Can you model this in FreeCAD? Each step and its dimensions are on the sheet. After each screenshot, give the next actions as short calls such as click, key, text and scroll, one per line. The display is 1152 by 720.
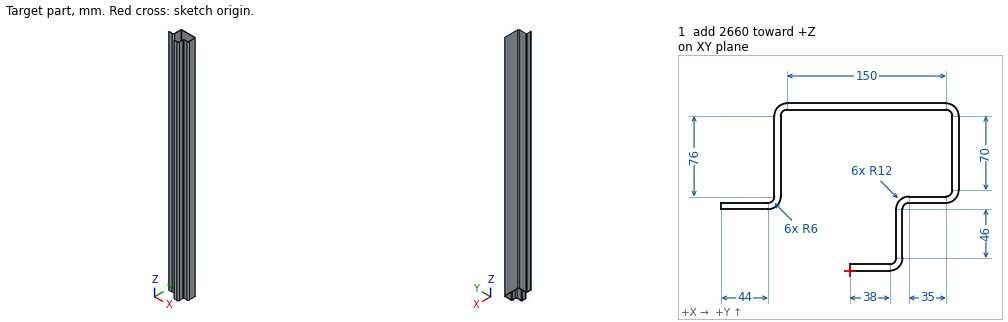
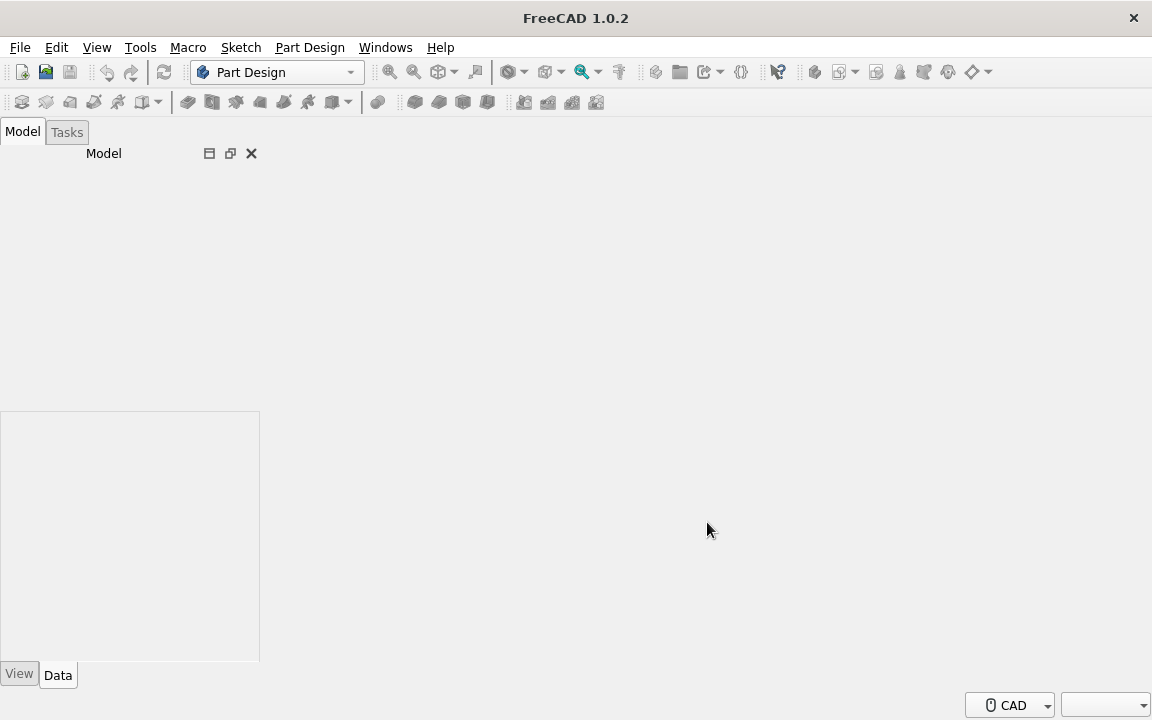
key(ctrl+n)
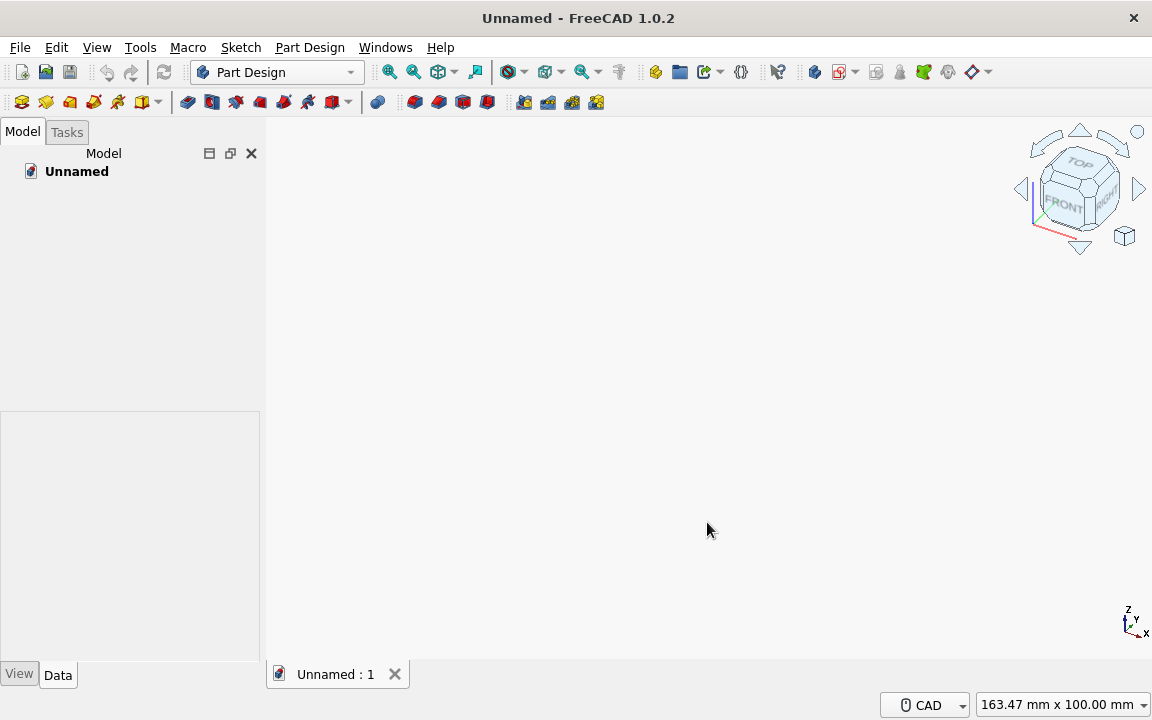
click(840, 72)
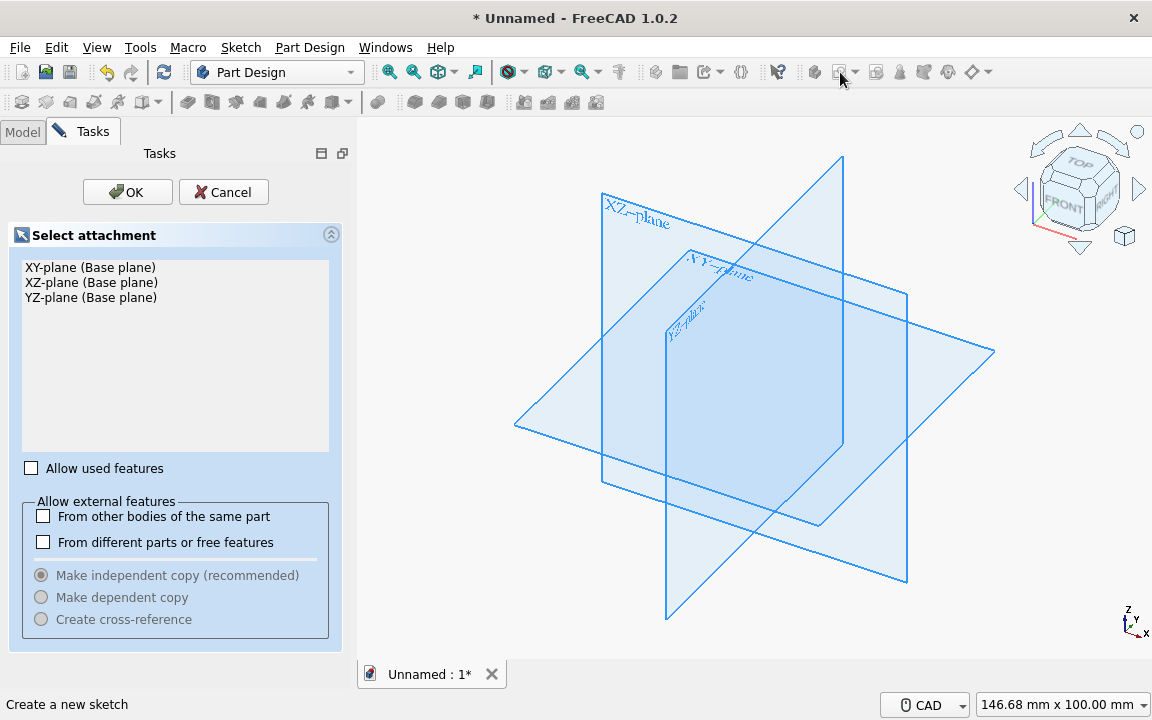
click(82, 268)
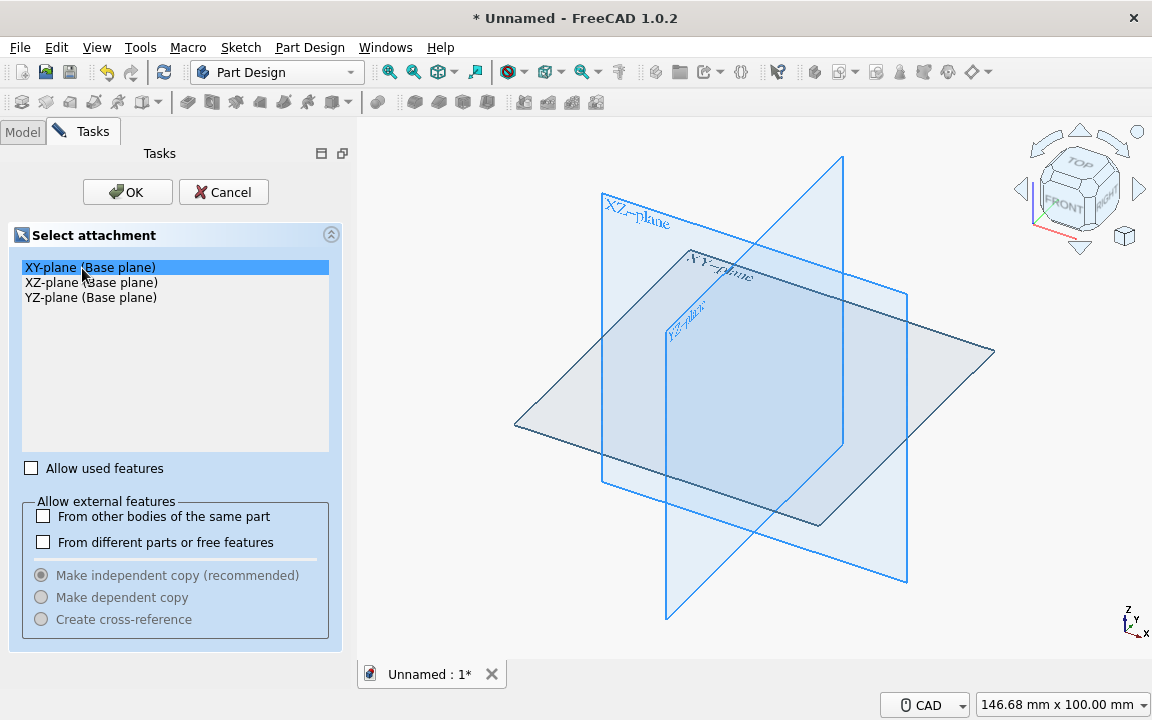
click(128, 192)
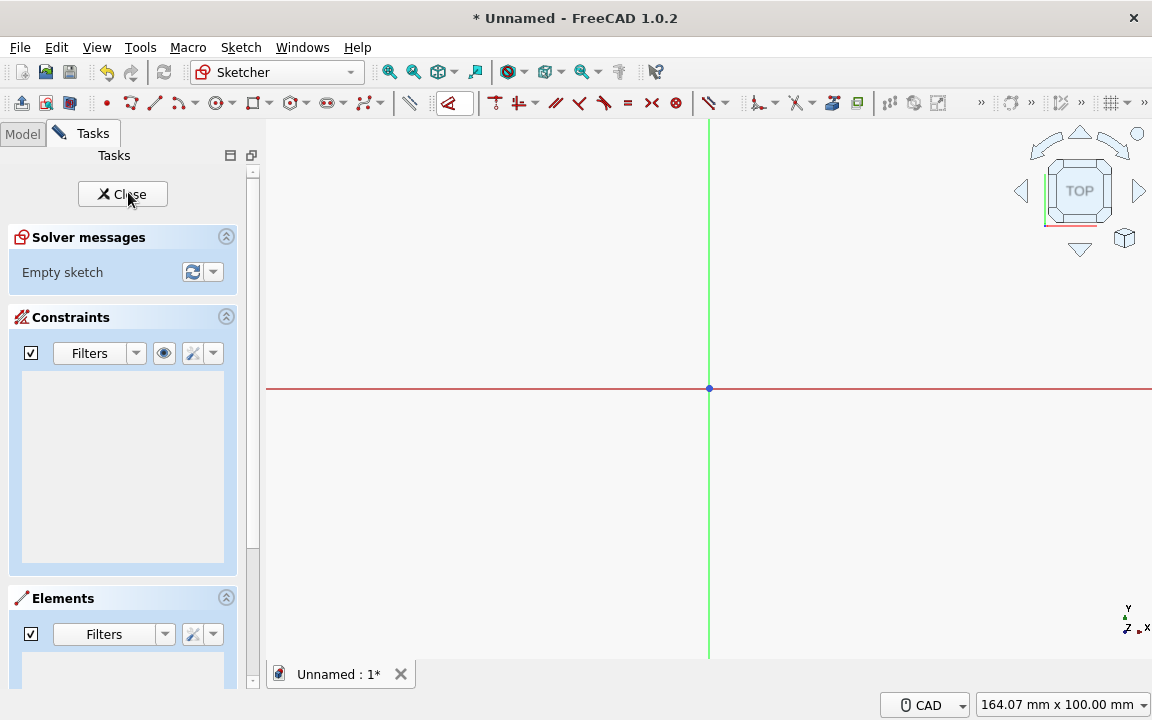
scroll(629, 631, down, 5)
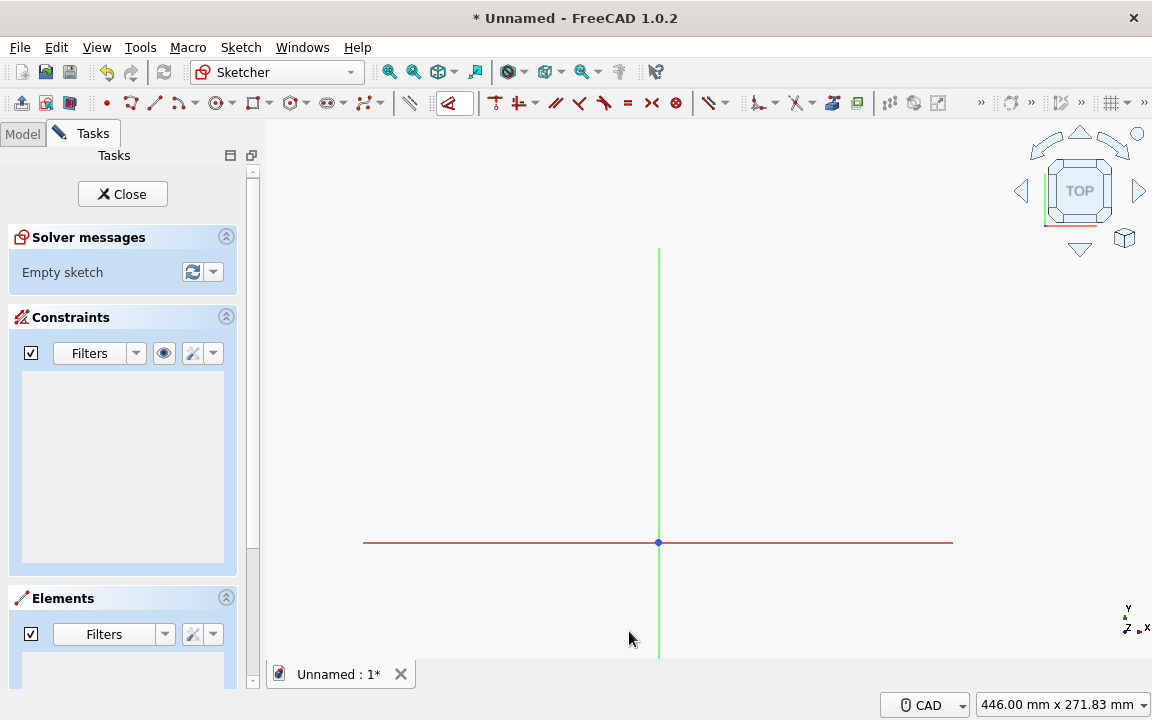
key(g)
key(l)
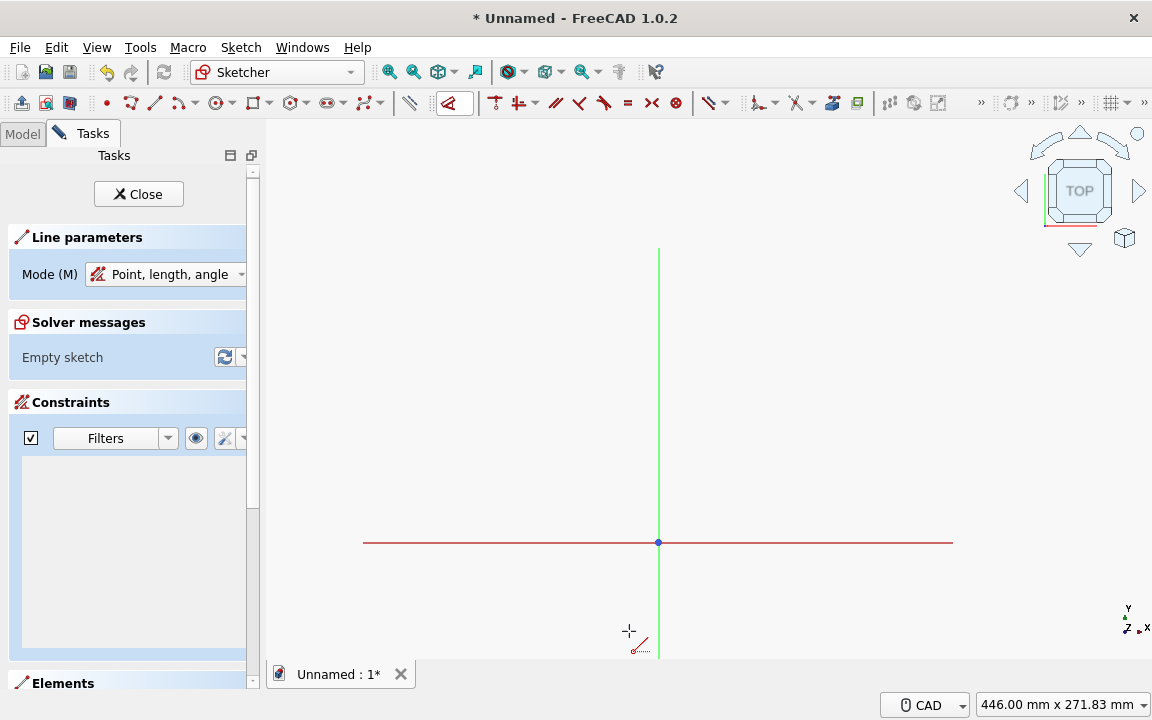
click(518, 253)
click(518, 404)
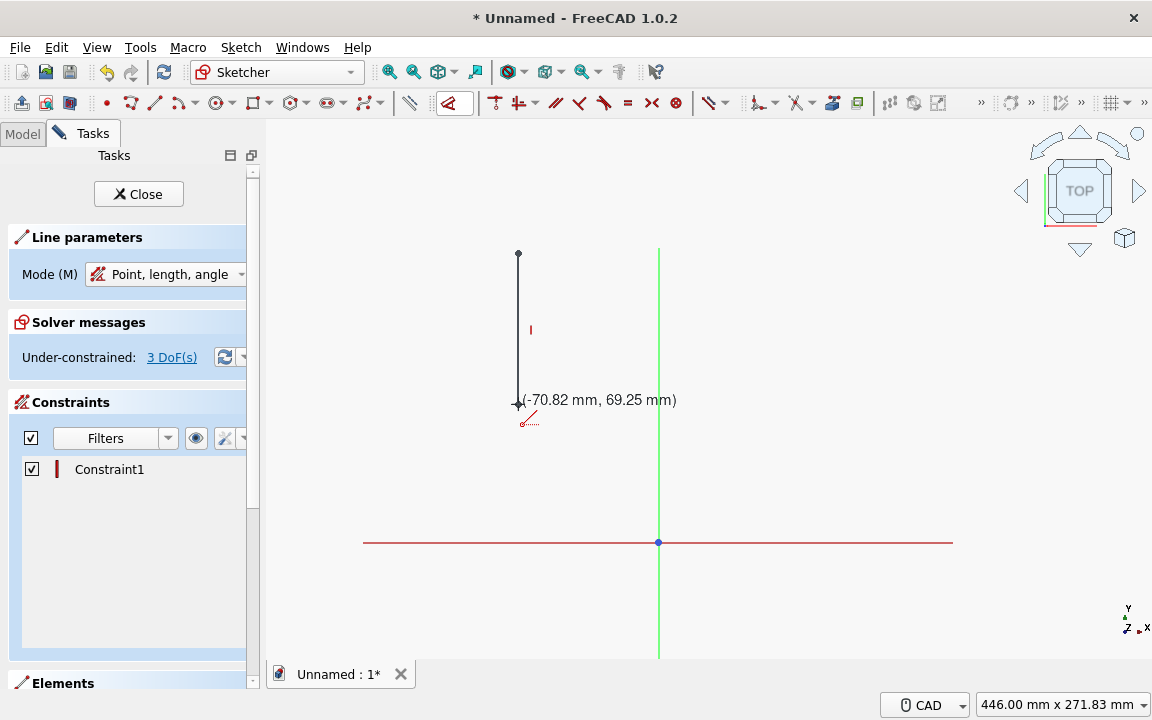
click(132, 104)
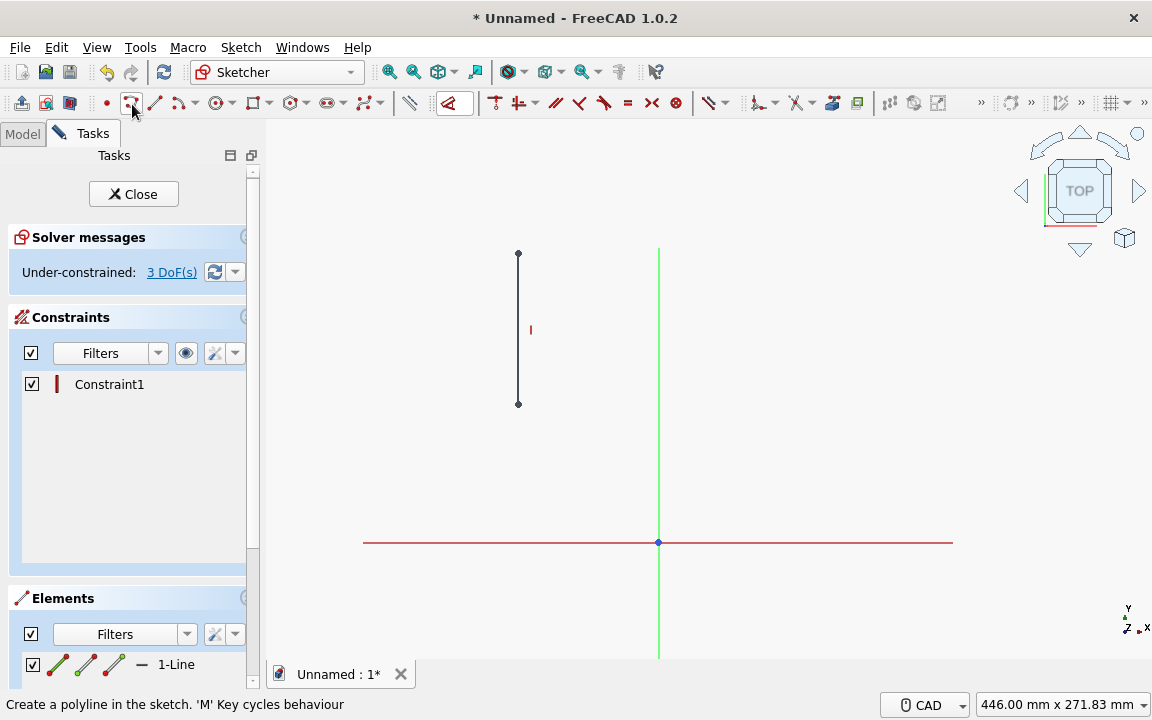
click(506, 415)
click(418, 415)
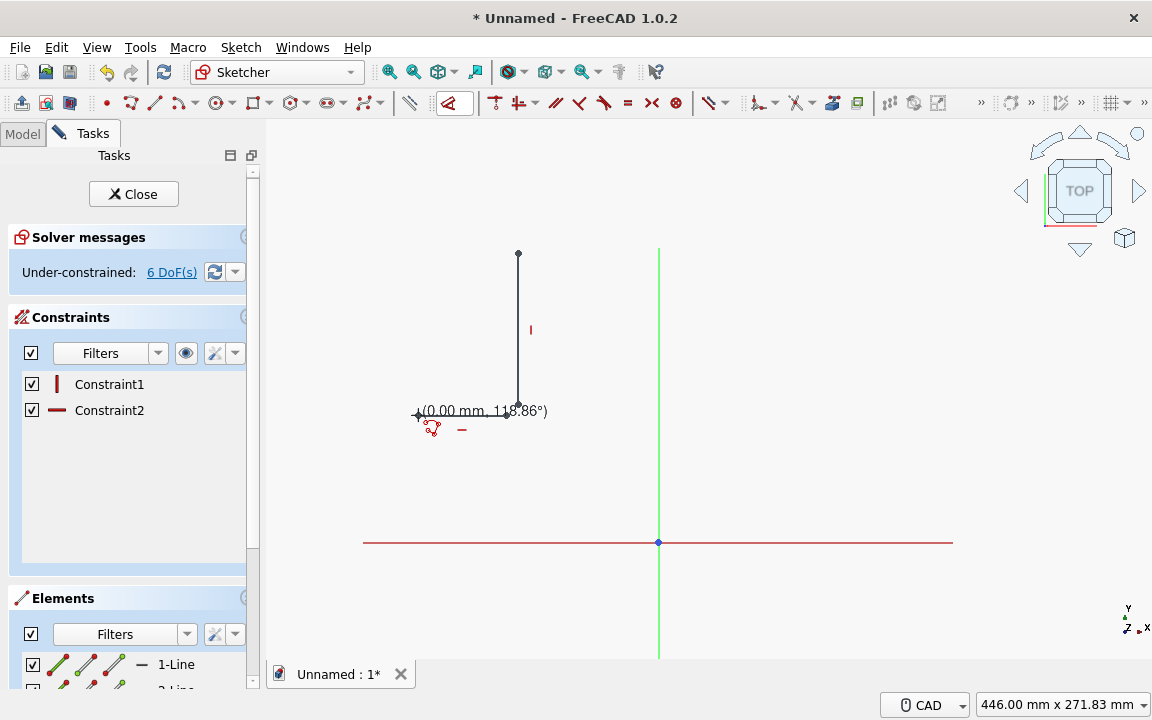
scroll(418, 427, up, 2)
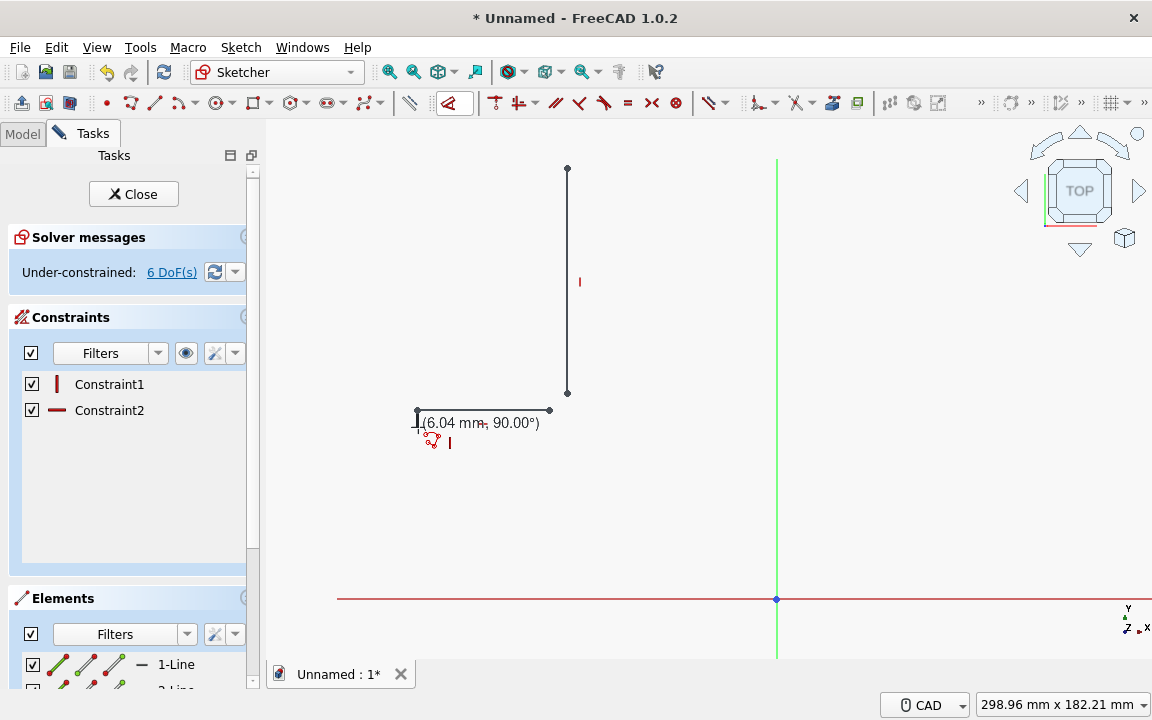
click(418, 427)
click(549, 427)
right_click(549, 427)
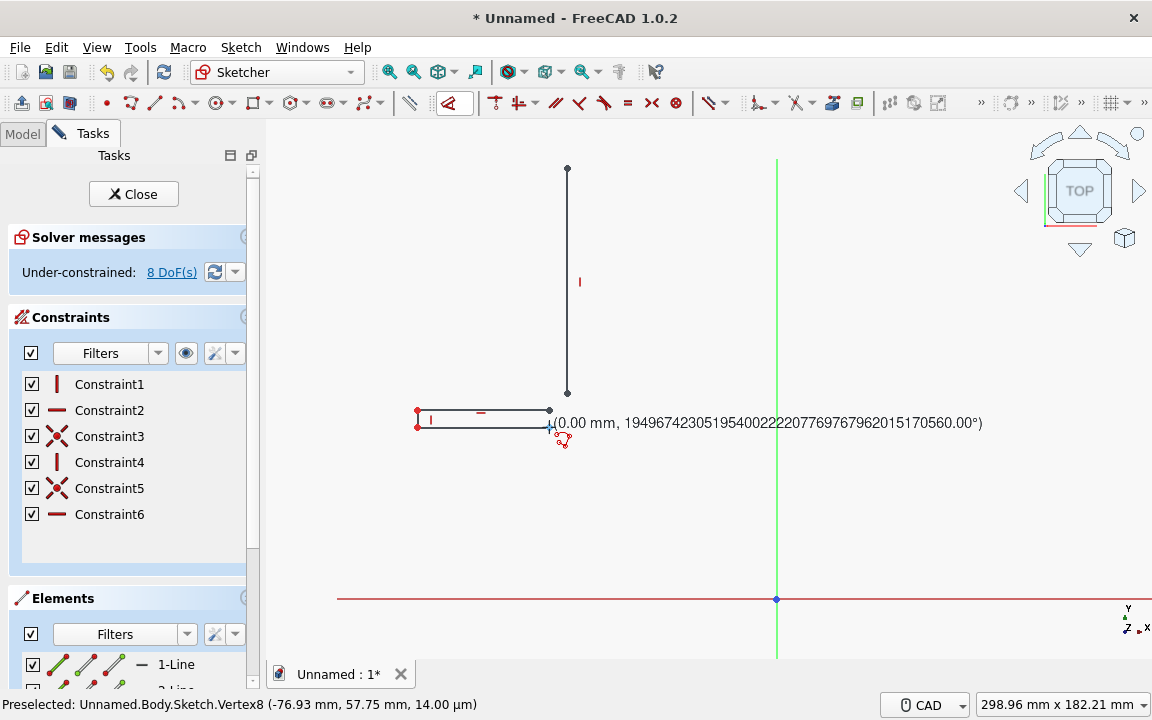
key(g)
key(l)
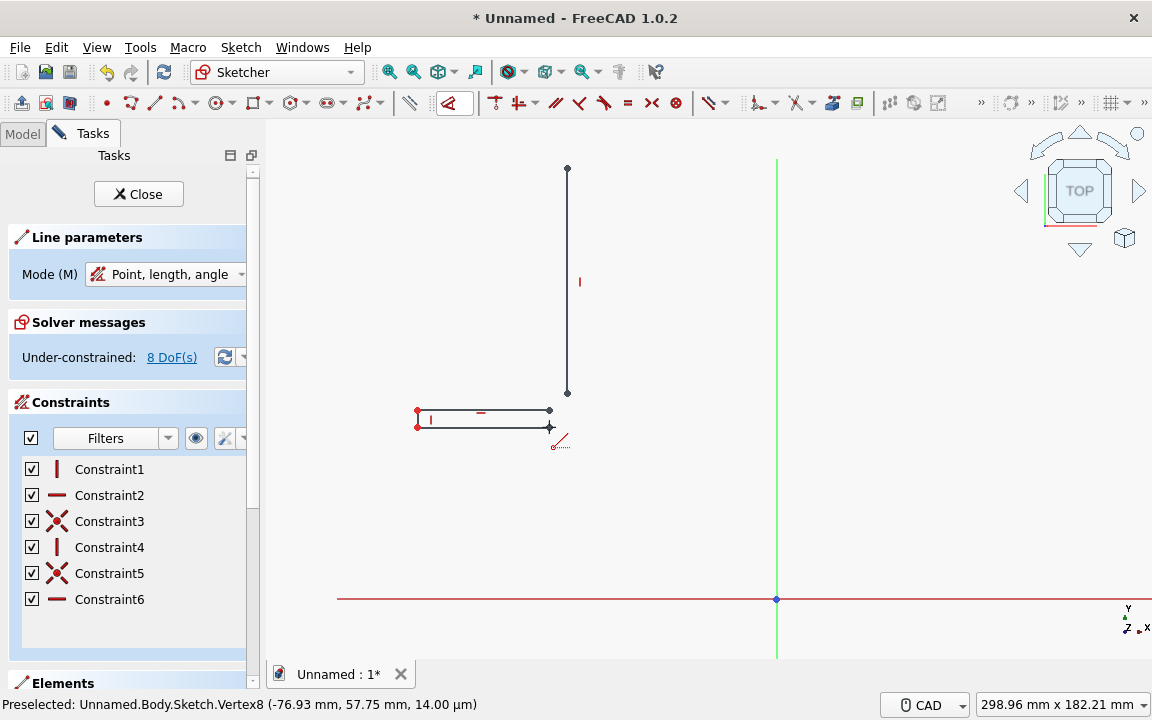
click(584, 392)
click(584, 166)